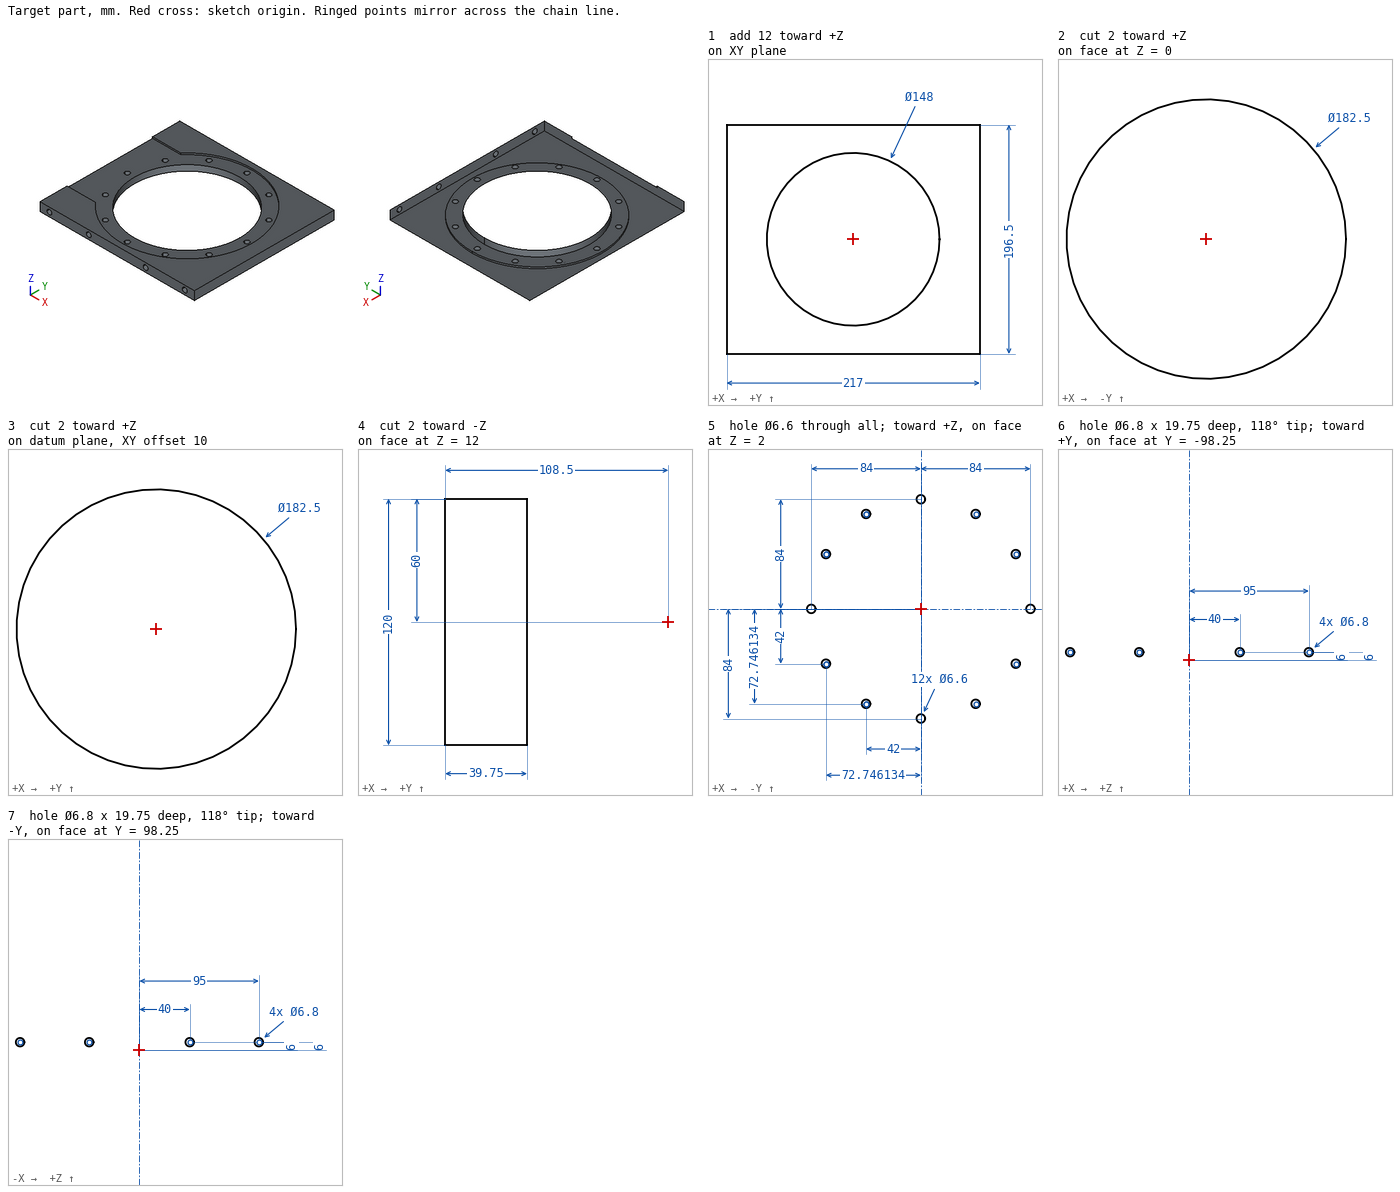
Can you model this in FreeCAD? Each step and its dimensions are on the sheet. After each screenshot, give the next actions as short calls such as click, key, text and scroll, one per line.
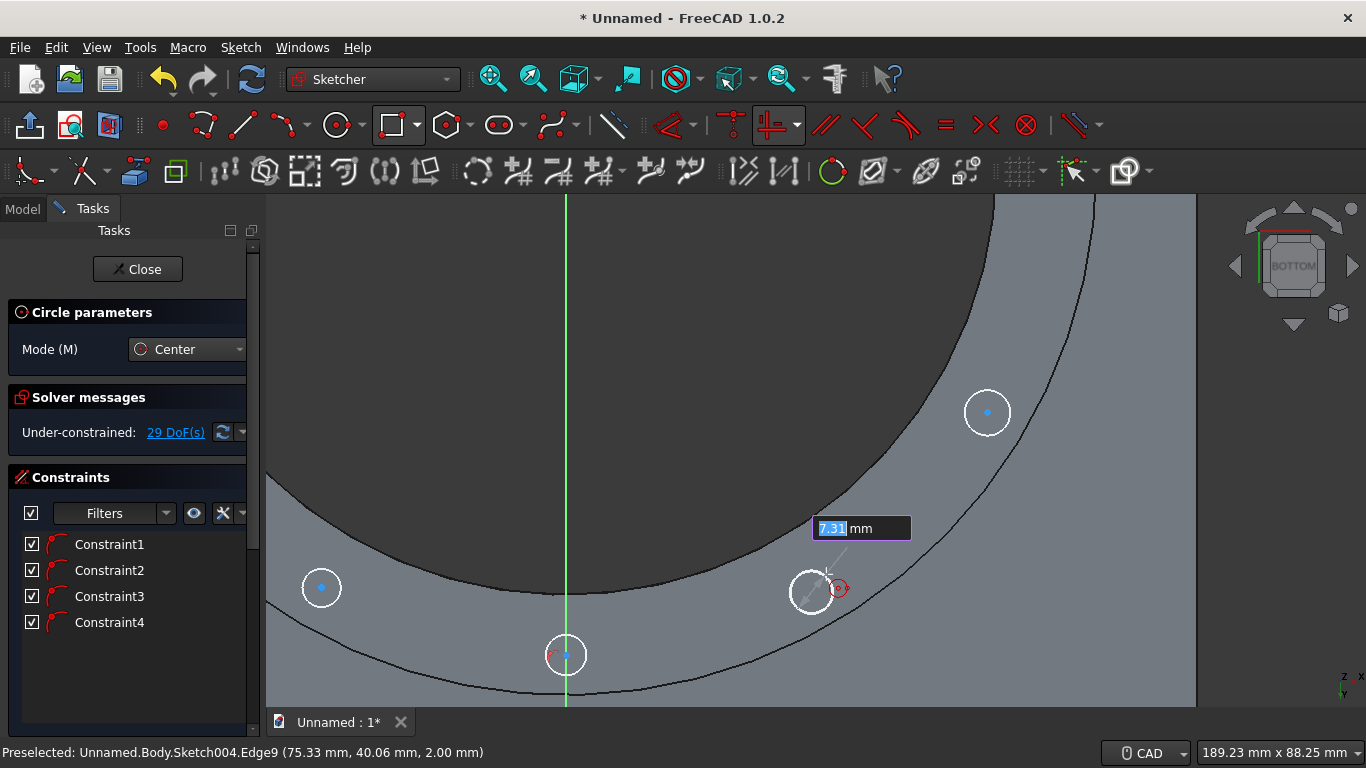
click(824, 574)
key(Escape)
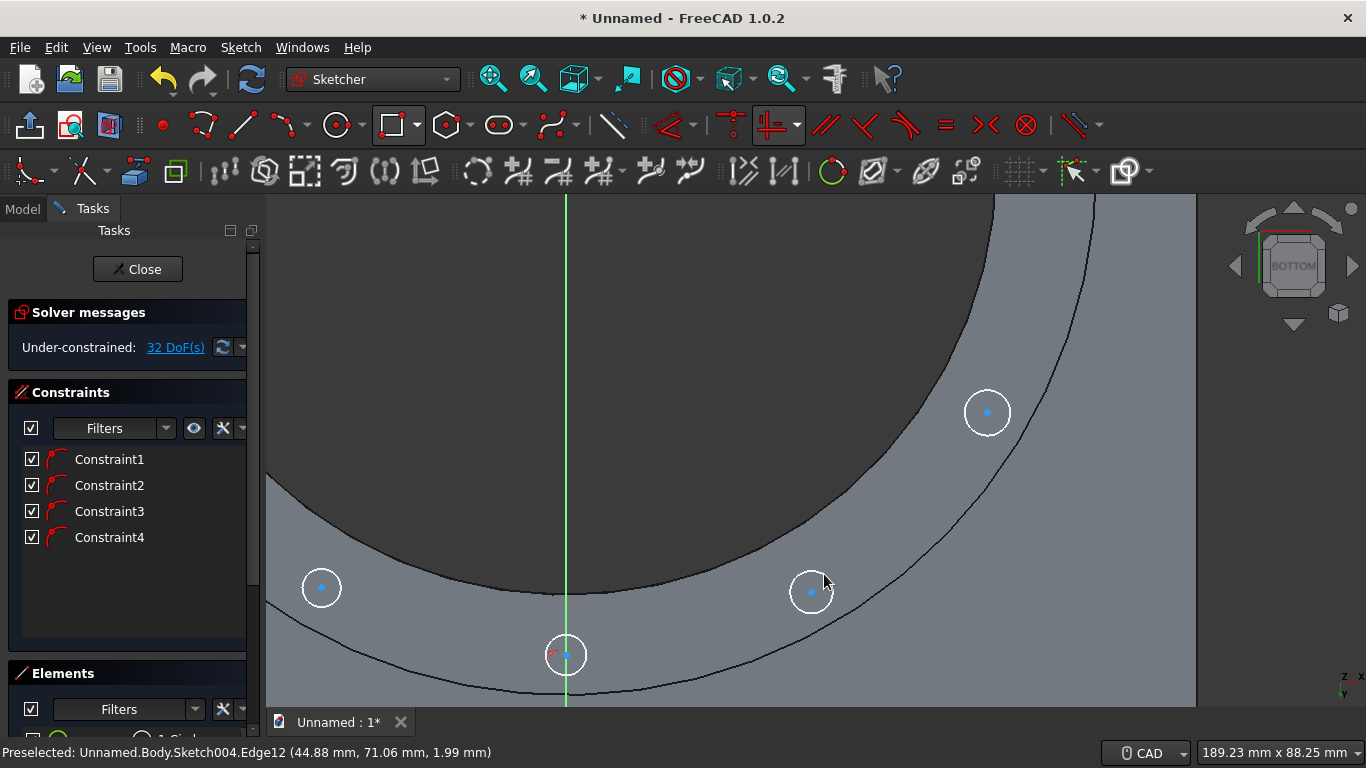
click(580, 641)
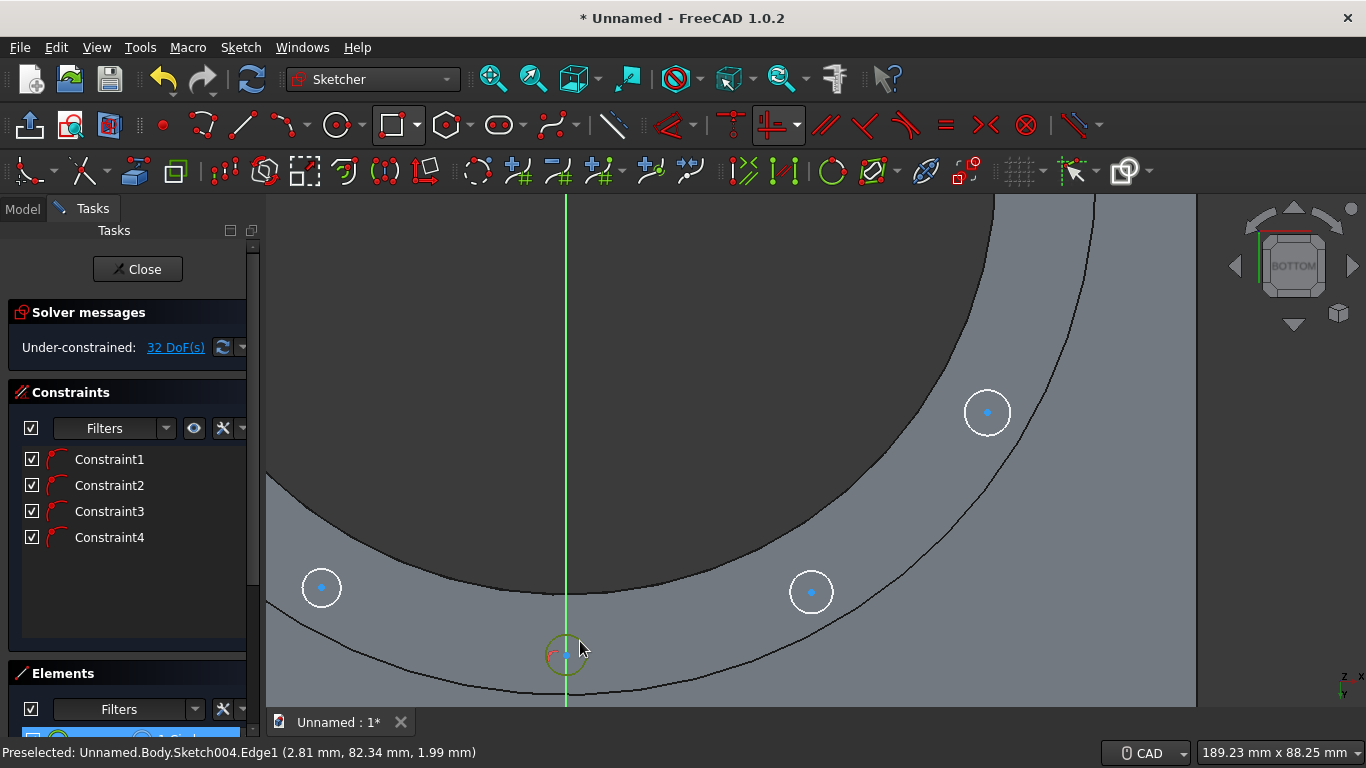
click(335, 574)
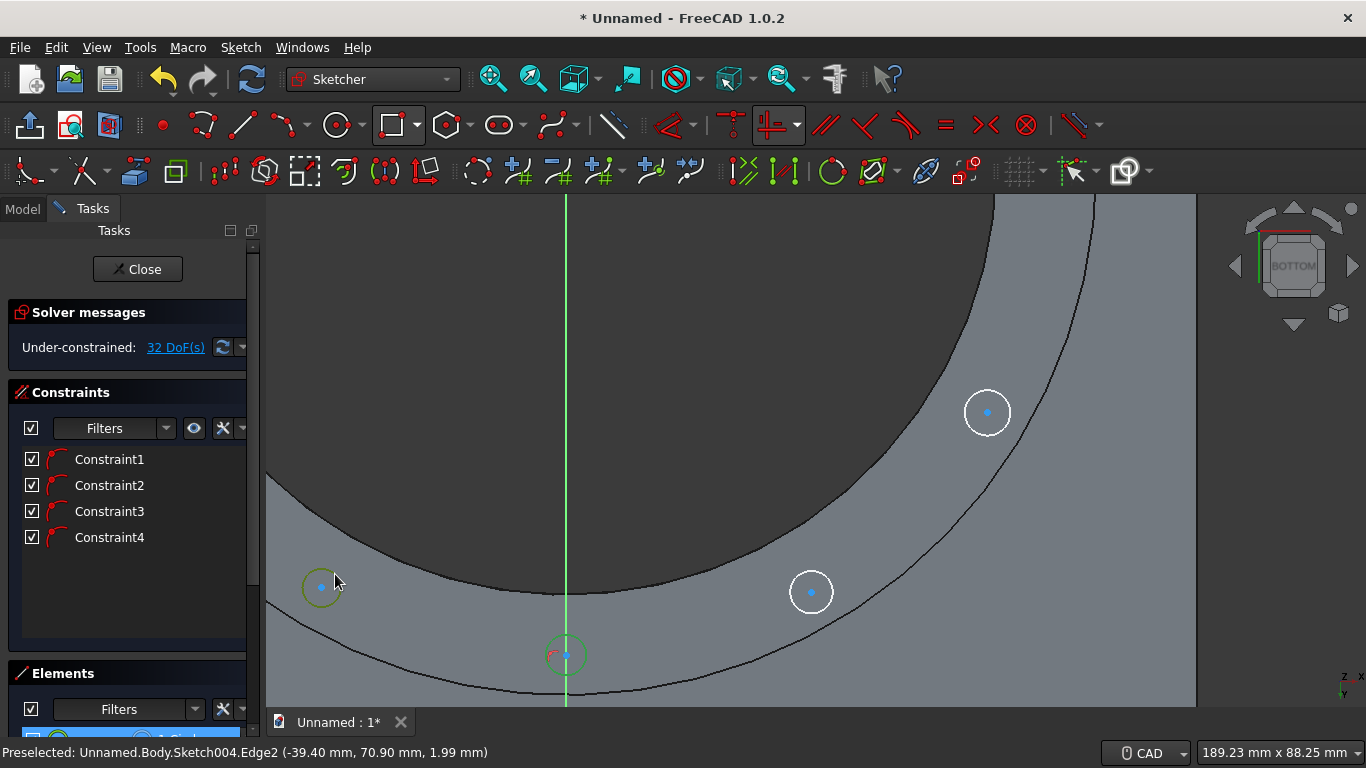
scroll(826, 574, down, 6)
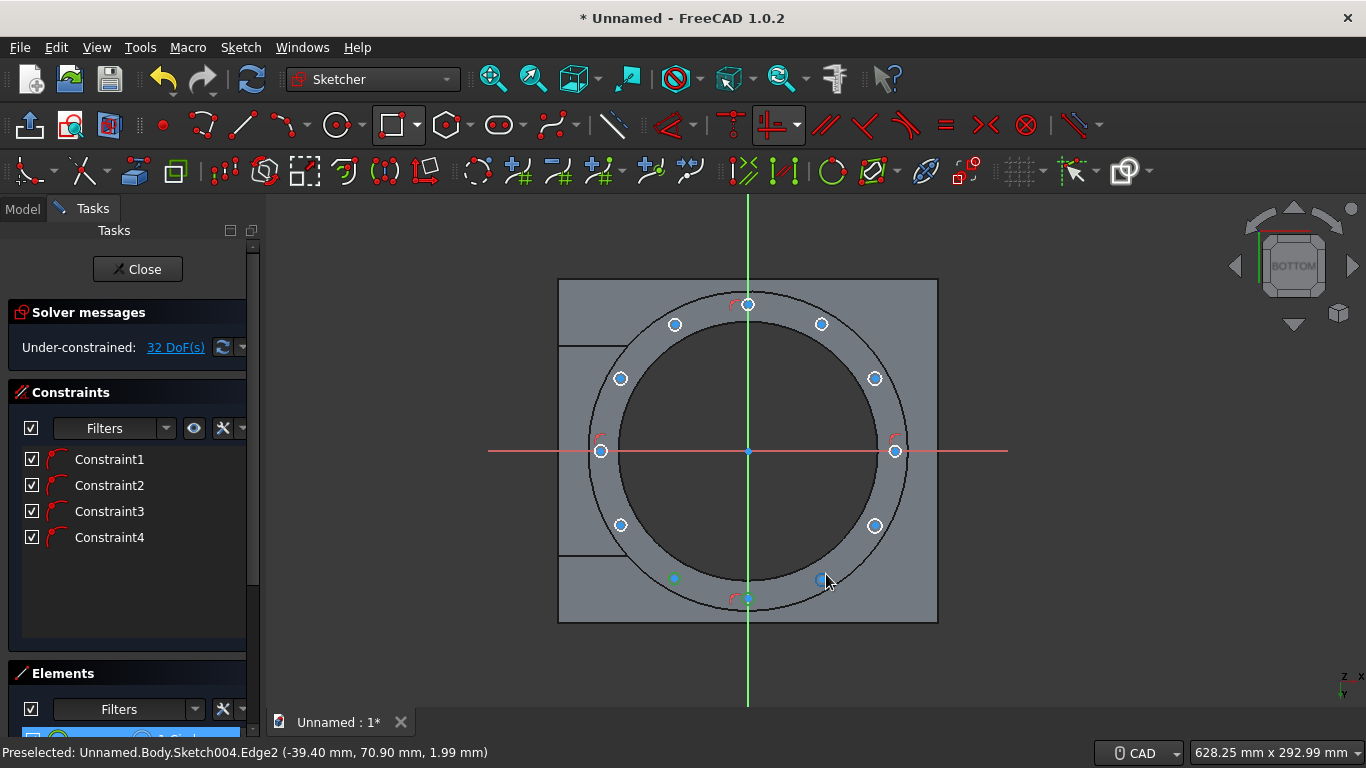
scroll(625, 521, up, 5)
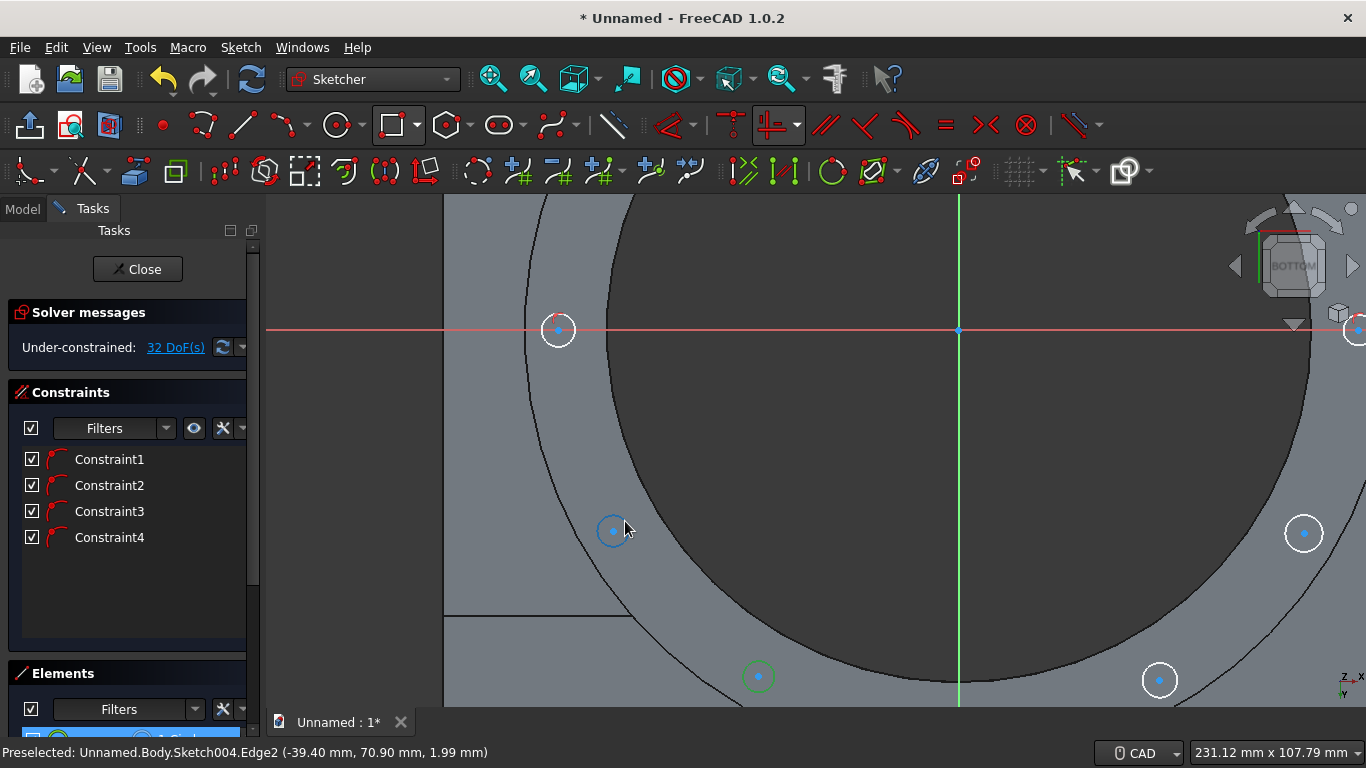
click(624, 520)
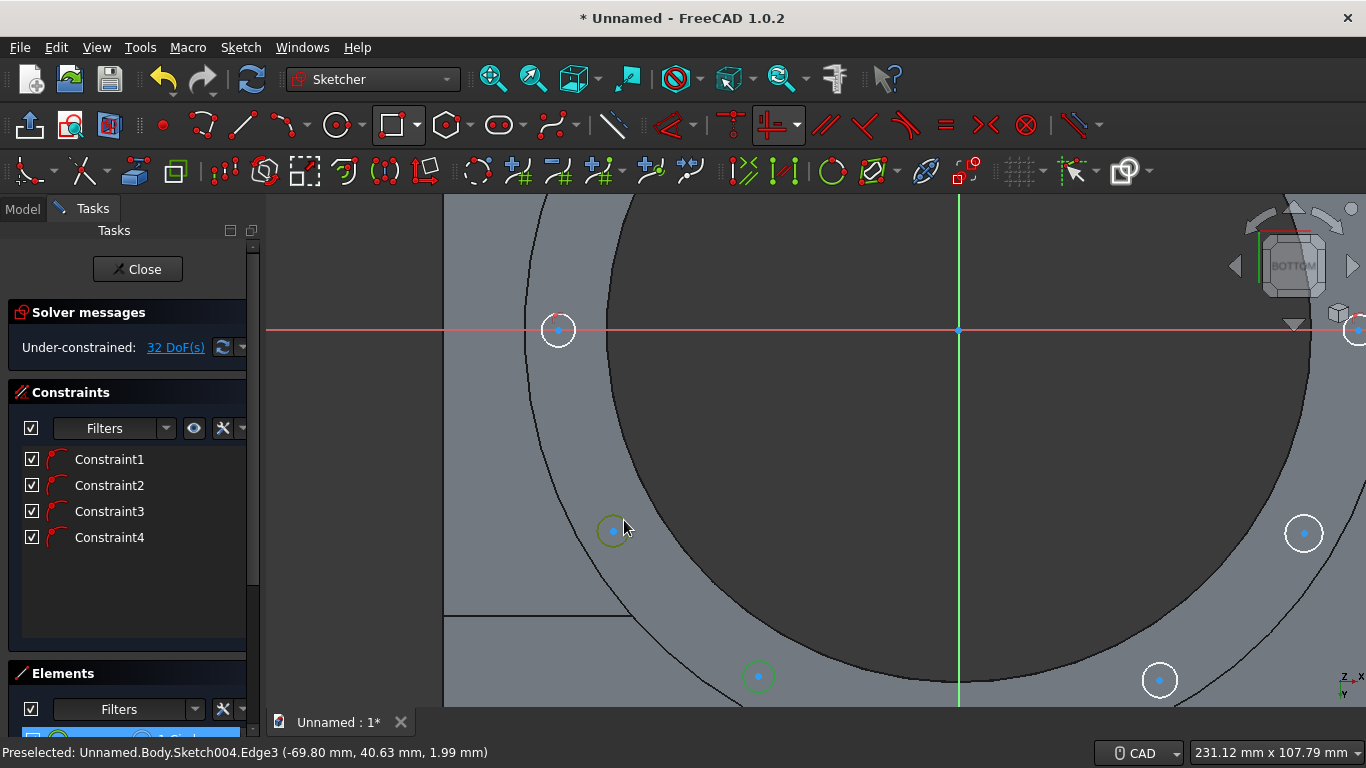
click(570, 318)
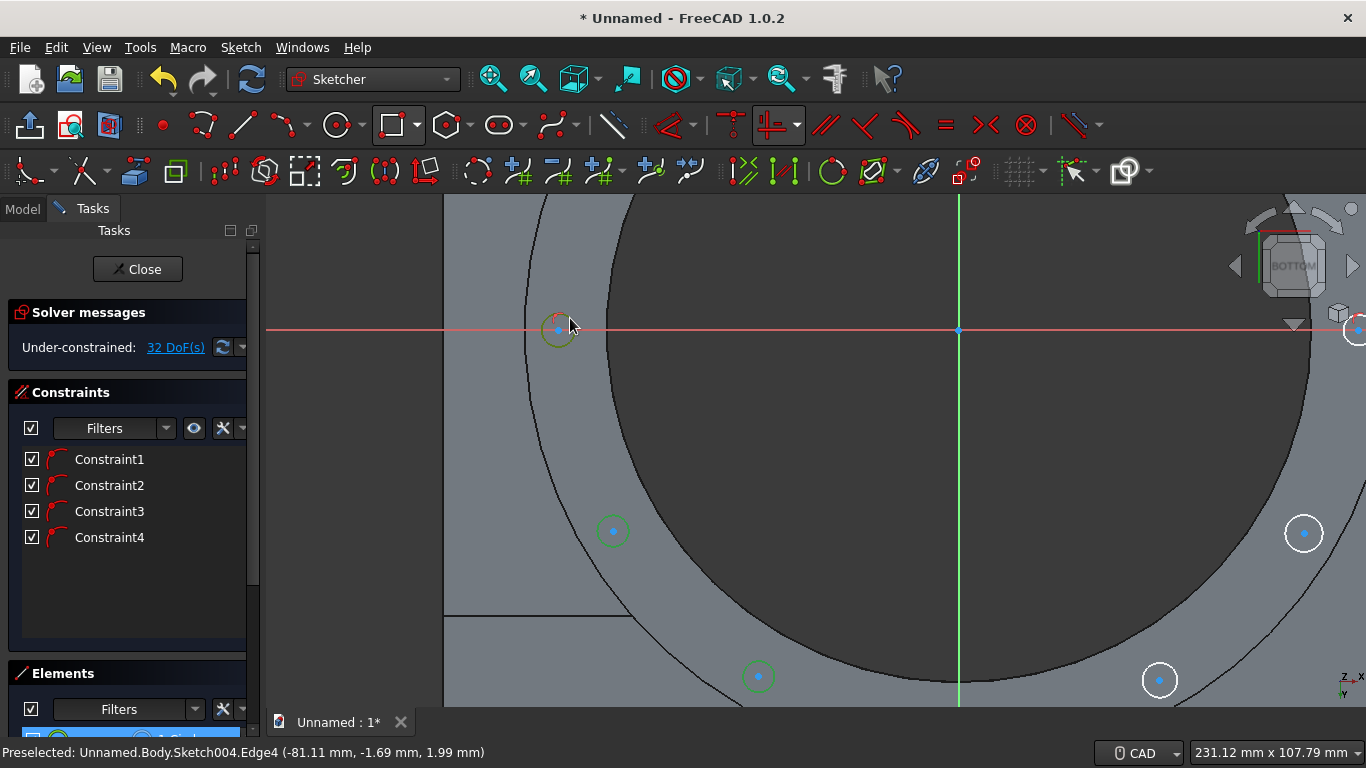
scroll(624, 521, down, 5)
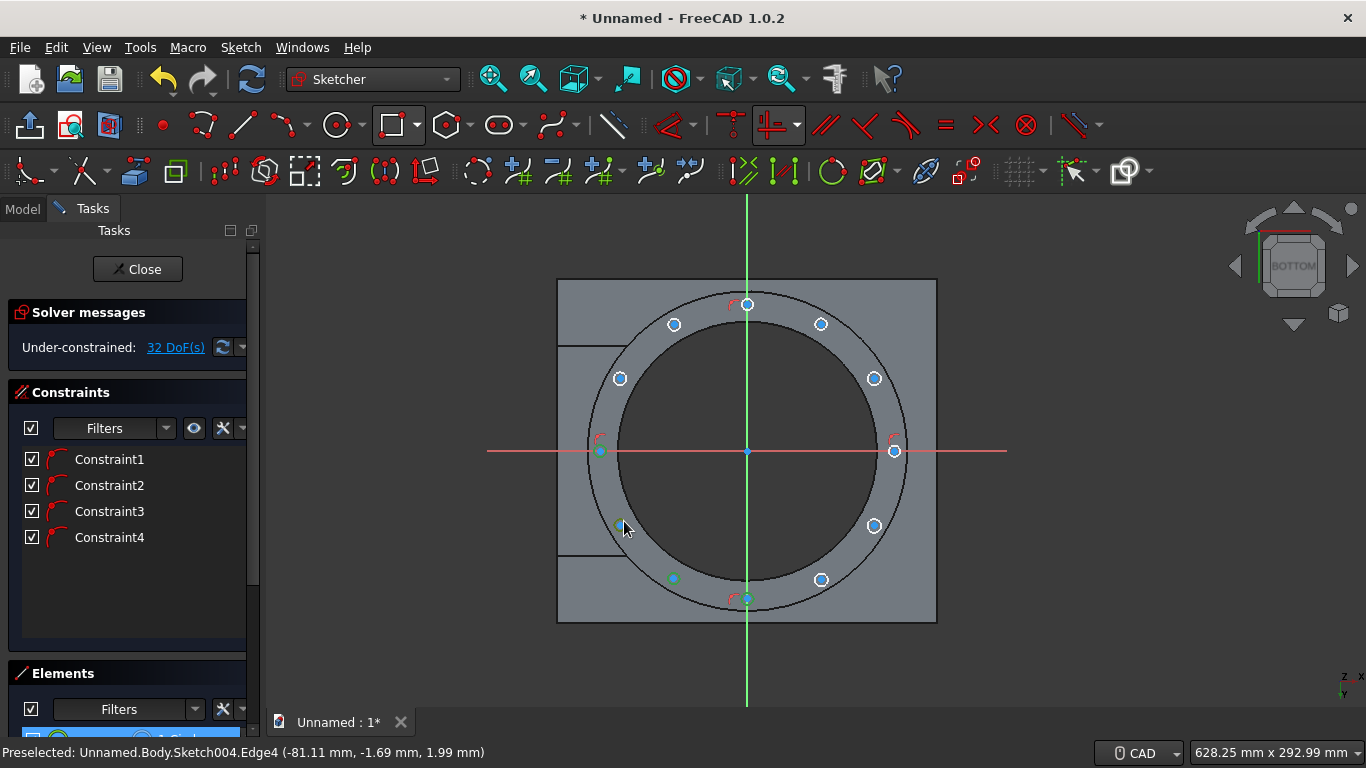
scroll(625, 374, up, 4)